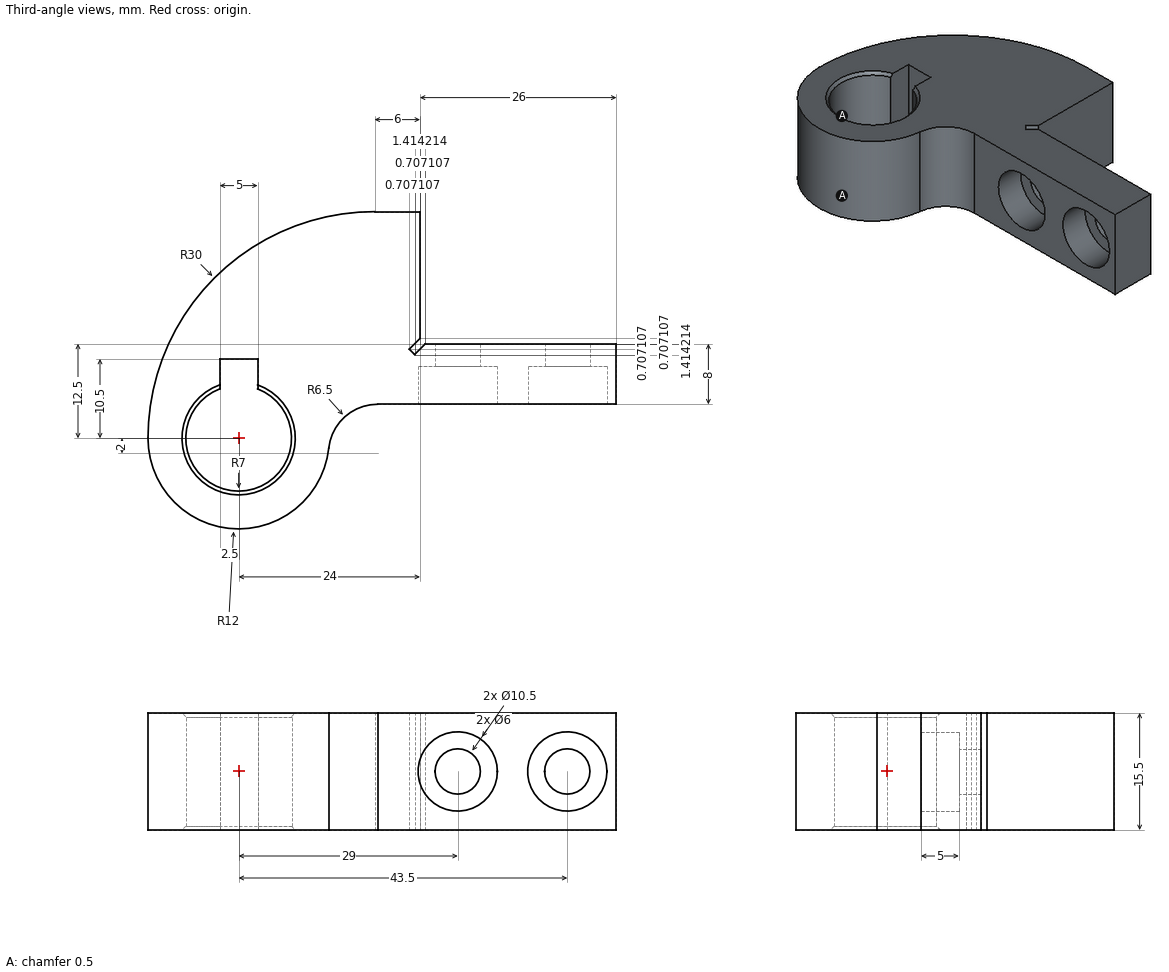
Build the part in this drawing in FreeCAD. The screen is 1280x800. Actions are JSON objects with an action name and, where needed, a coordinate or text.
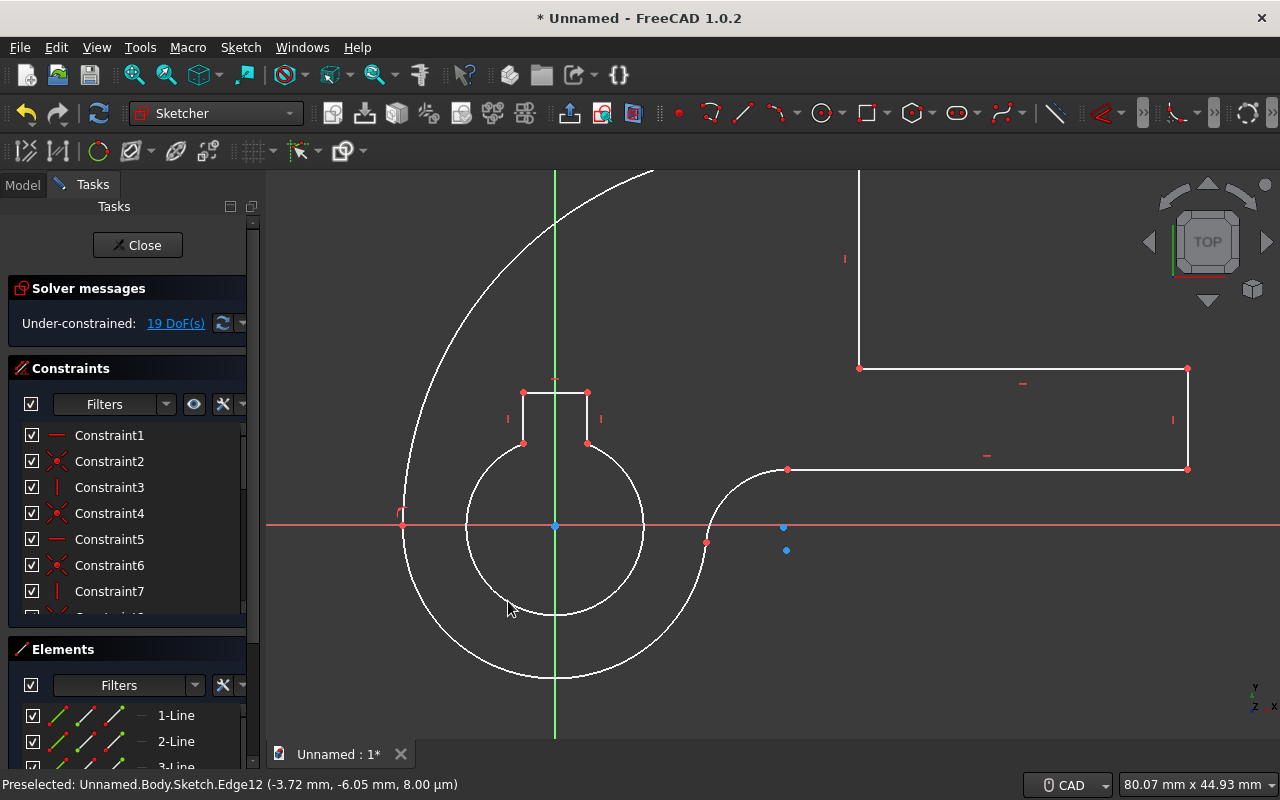
{"action": "left_click", "coordinate": [908, 470]}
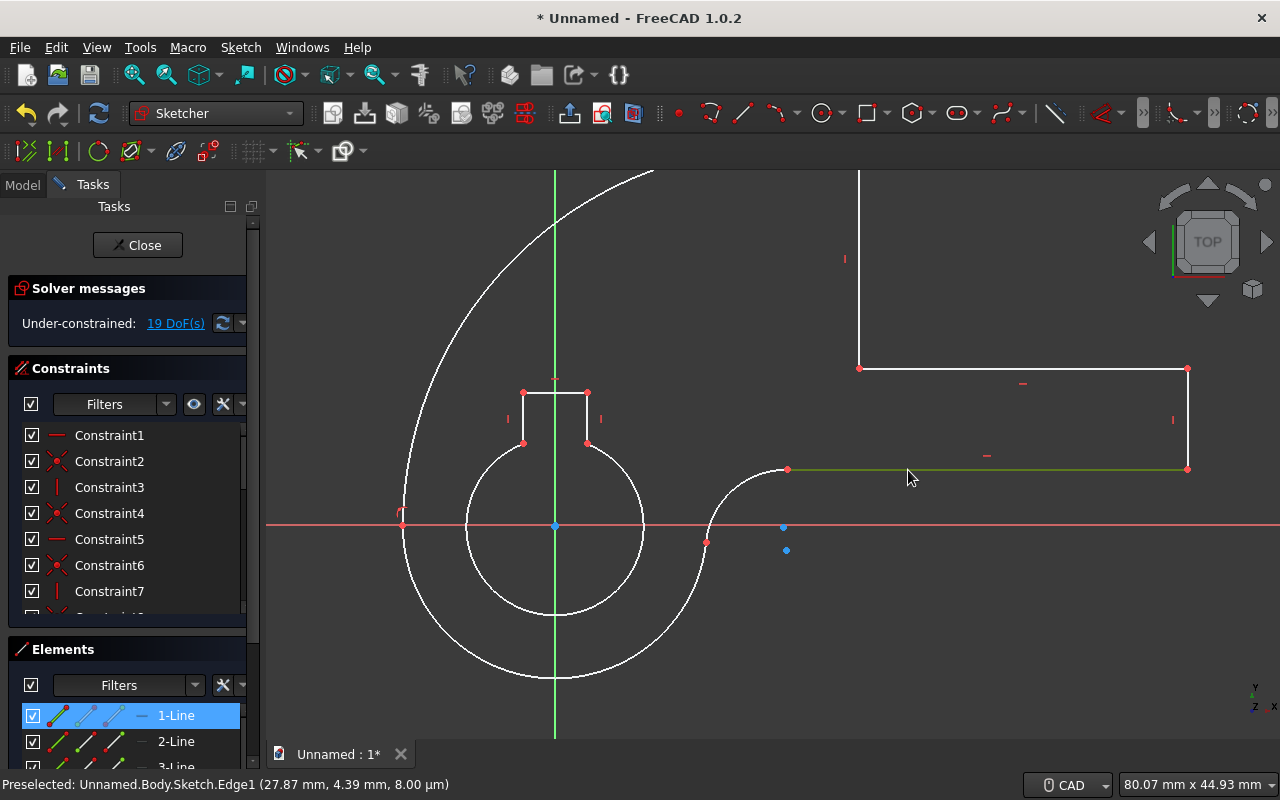
{"action": "left_click", "coordinate": [753, 477]}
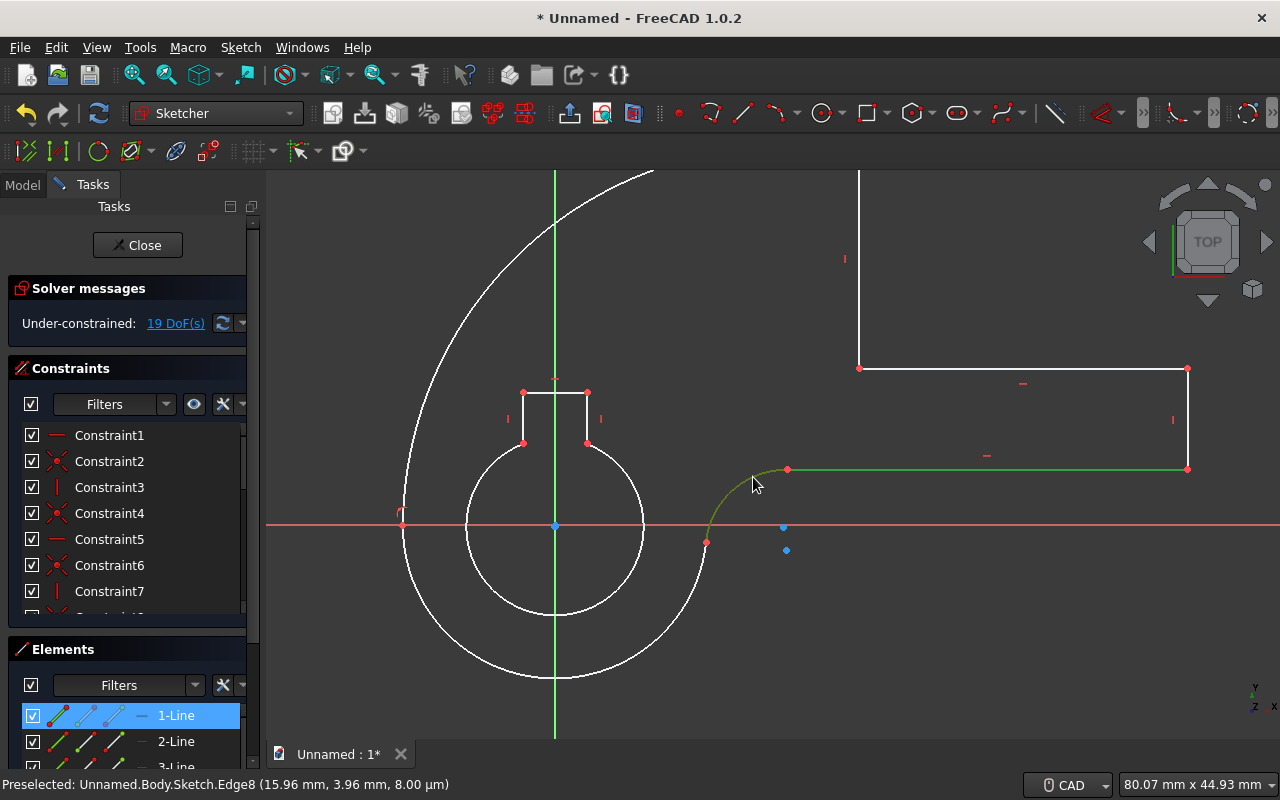
{"action": "key", "text": "t"}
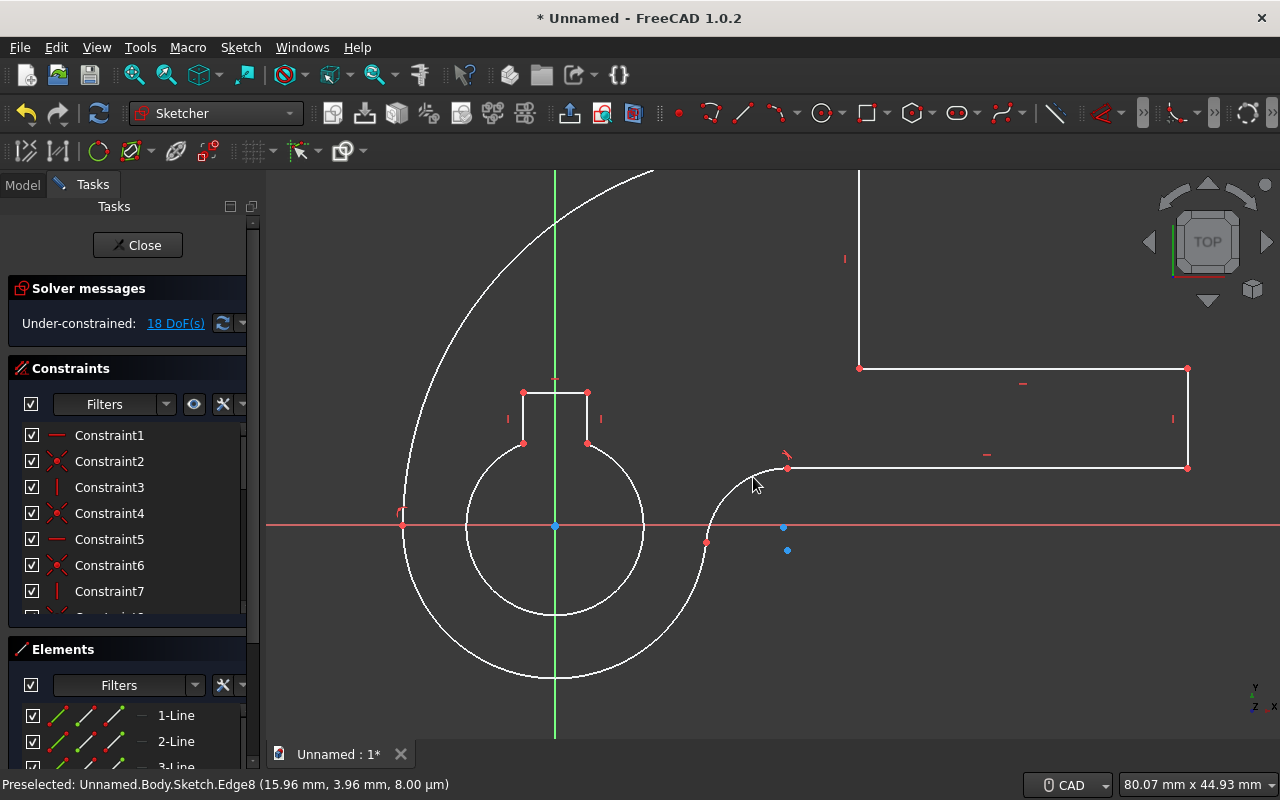
{"action": "scroll", "coordinate": [519, 542], "scroll_direction": "down", "scroll_amount": 2}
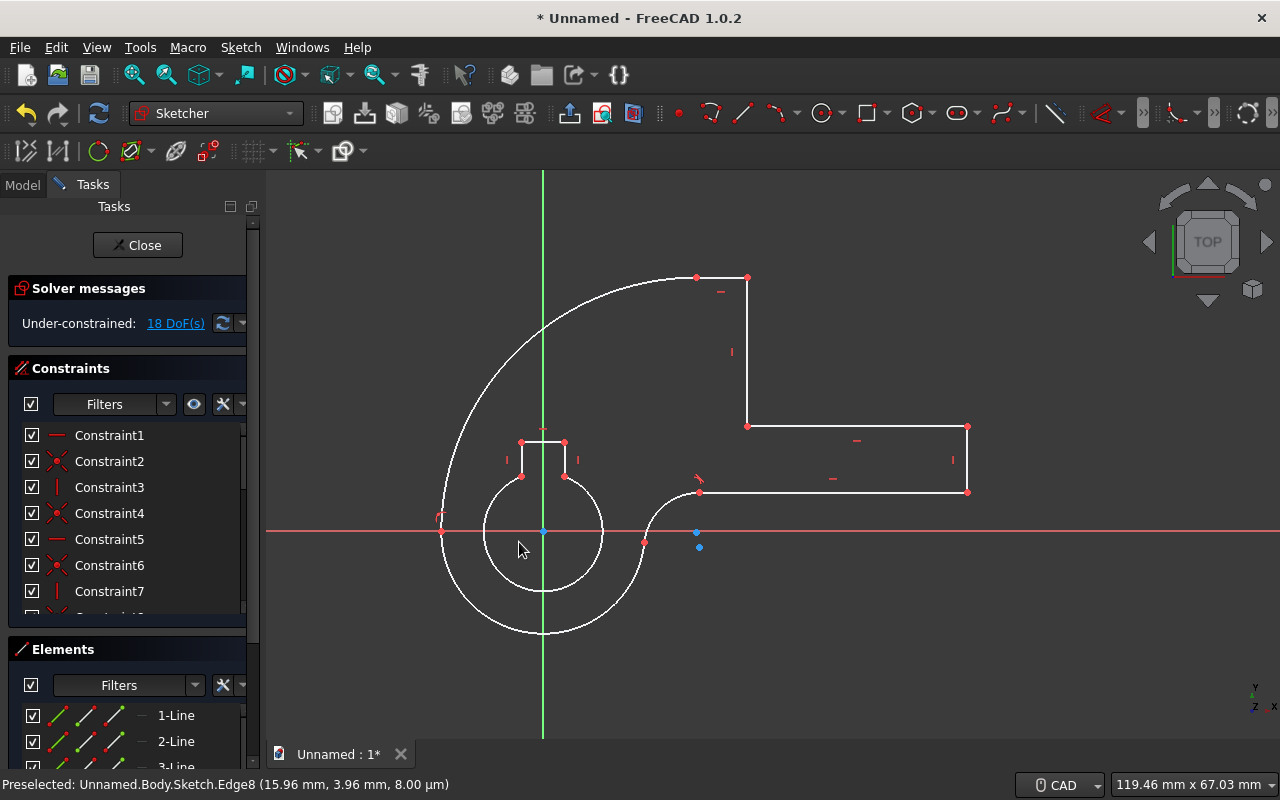
{"action": "left_click", "coordinate": [732, 278]}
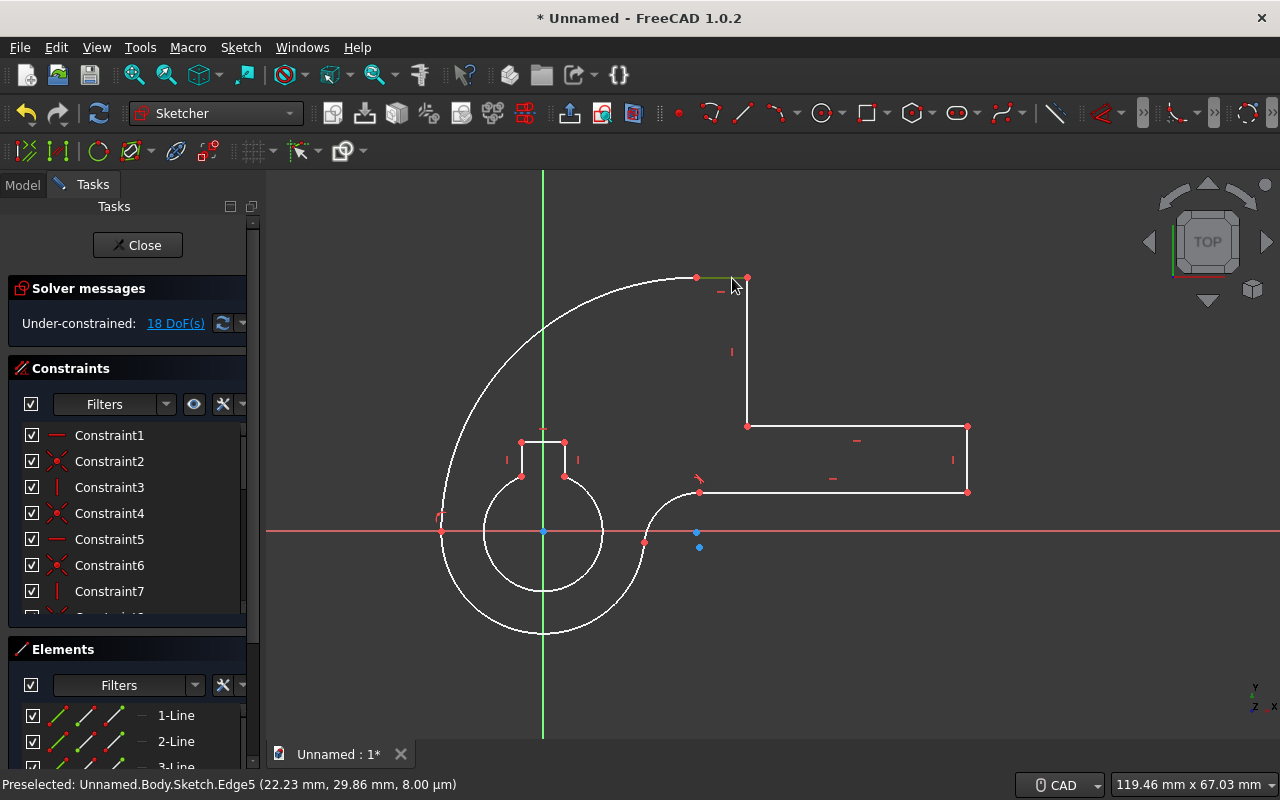
{"action": "left_click", "coordinate": [581, 305]}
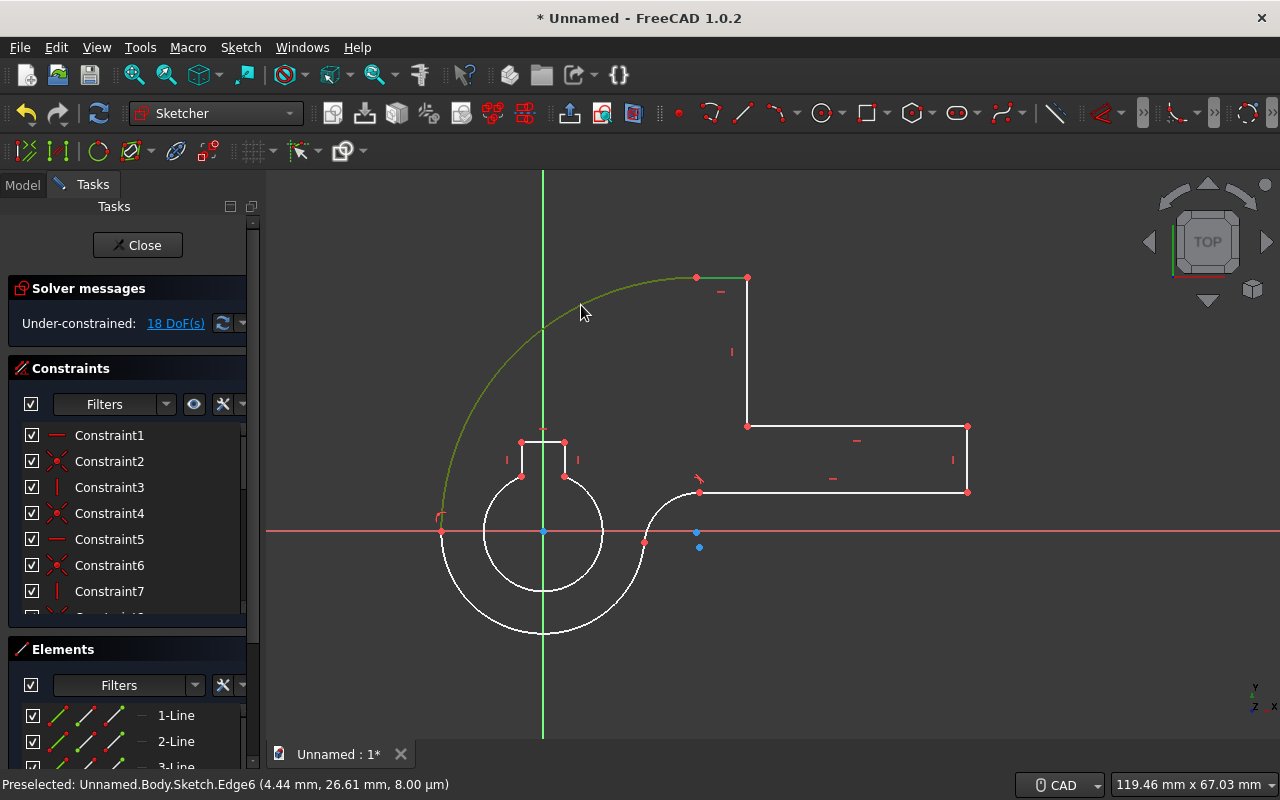
{"action": "key", "text": "t"}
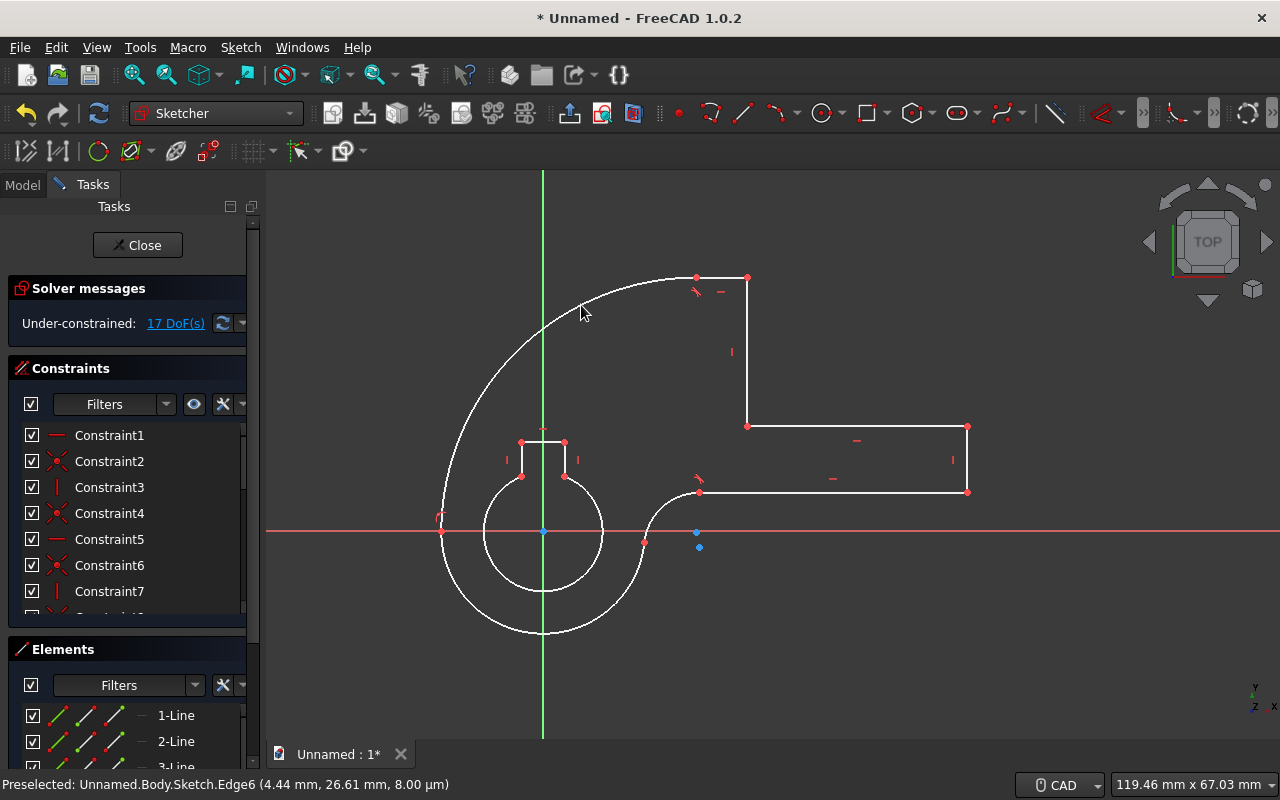
{"action": "left_click", "coordinate": [581, 305]}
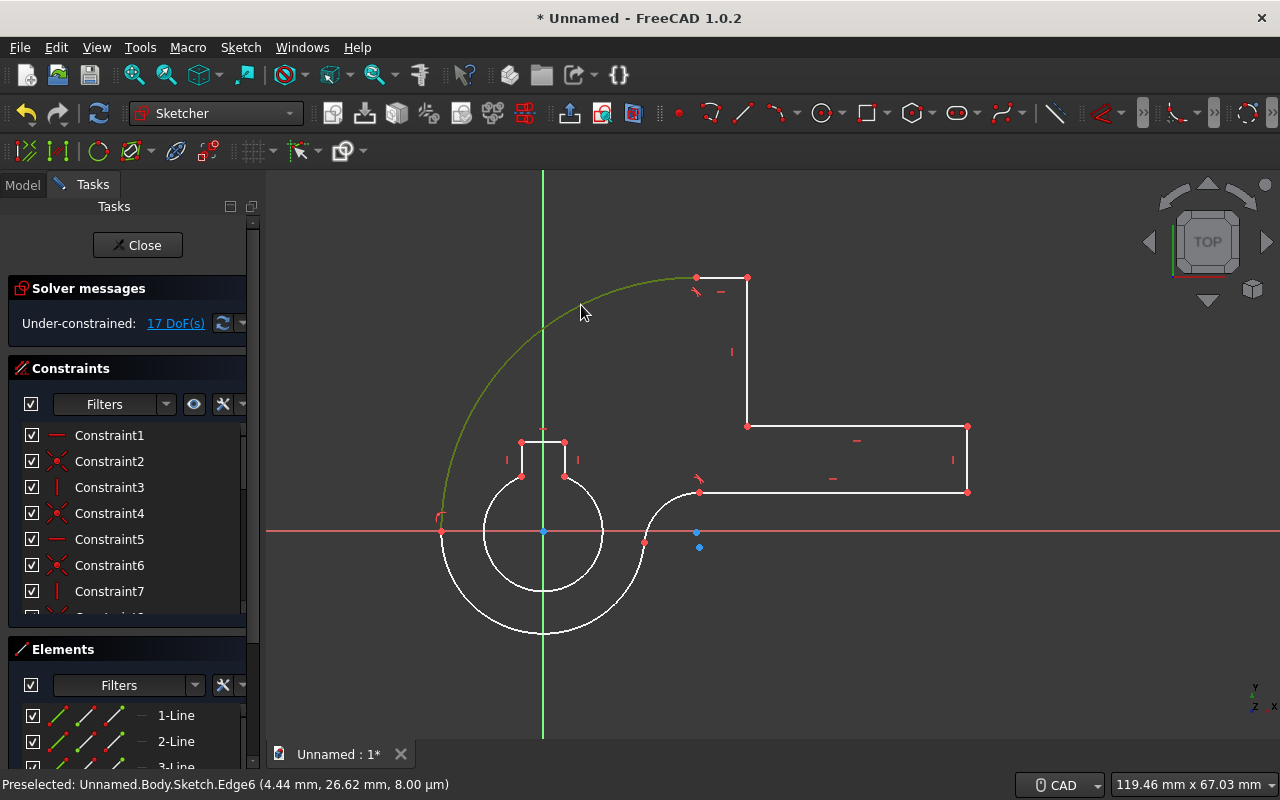
{"action": "left_click", "coordinate": [480, 612]}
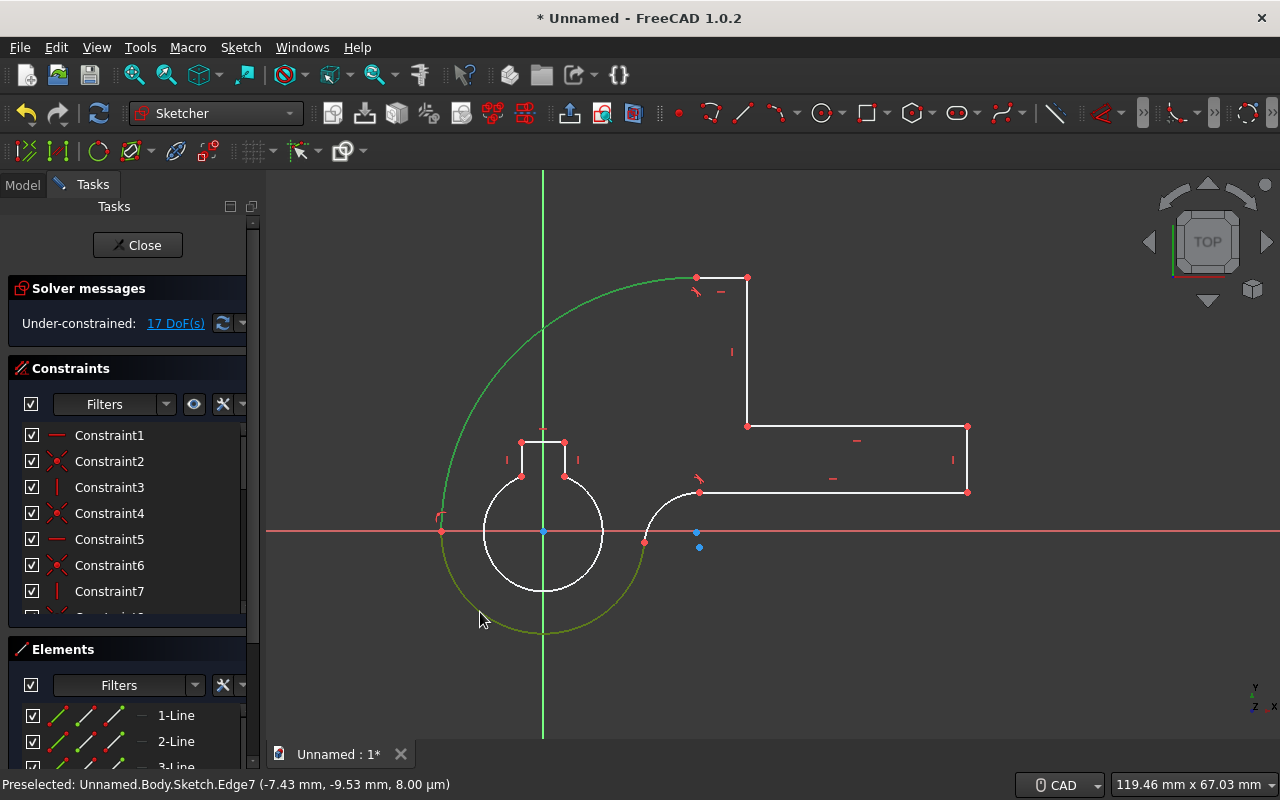
{"action": "key", "text": "t"}